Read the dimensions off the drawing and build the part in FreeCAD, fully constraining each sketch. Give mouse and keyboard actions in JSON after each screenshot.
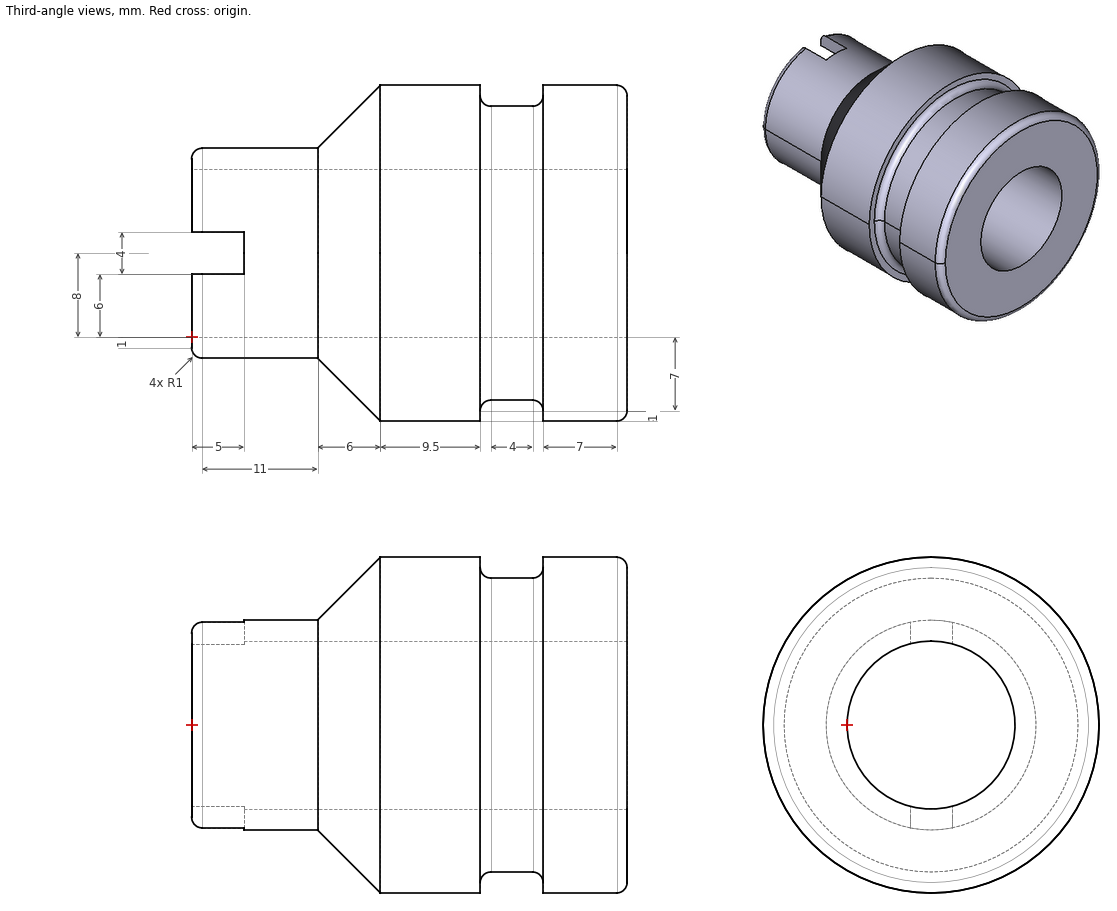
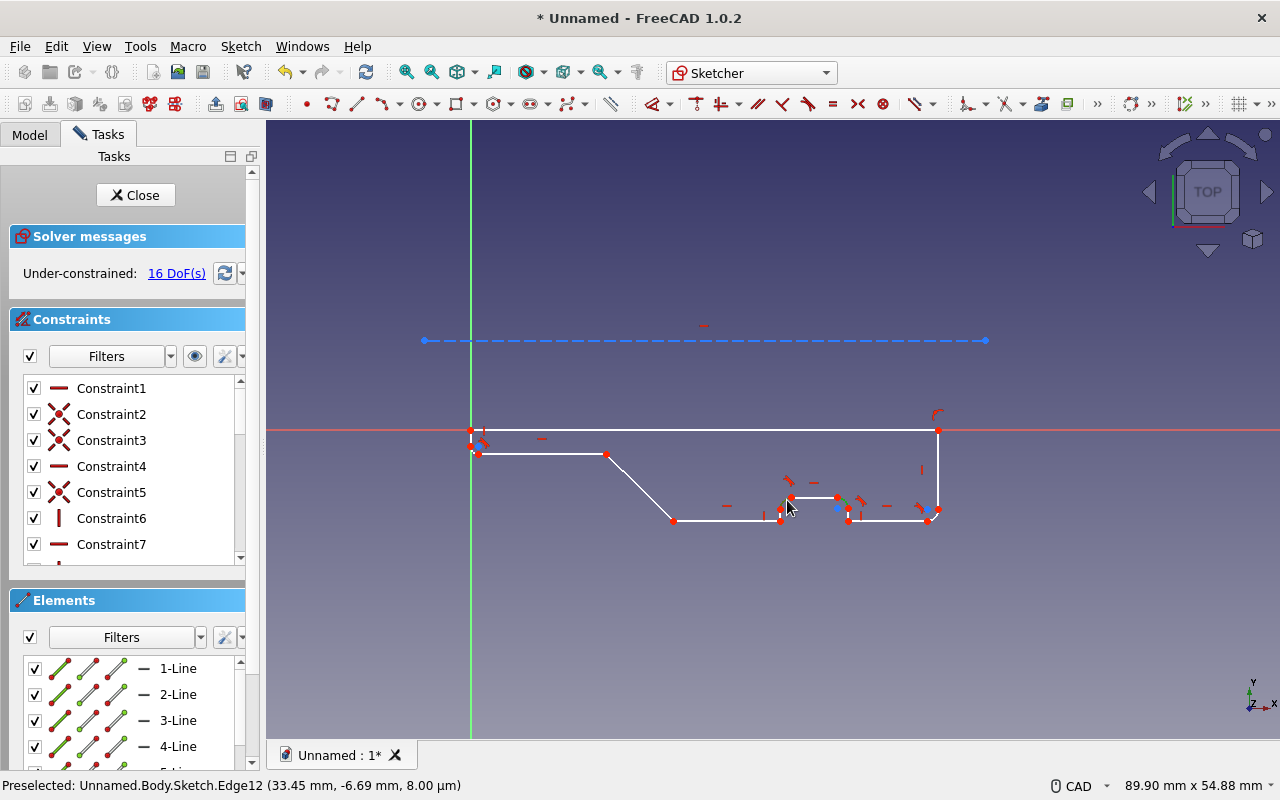
{"action": "scroll", "coordinate": [932, 520], "scroll_direction": "up", "scroll_amount": 5}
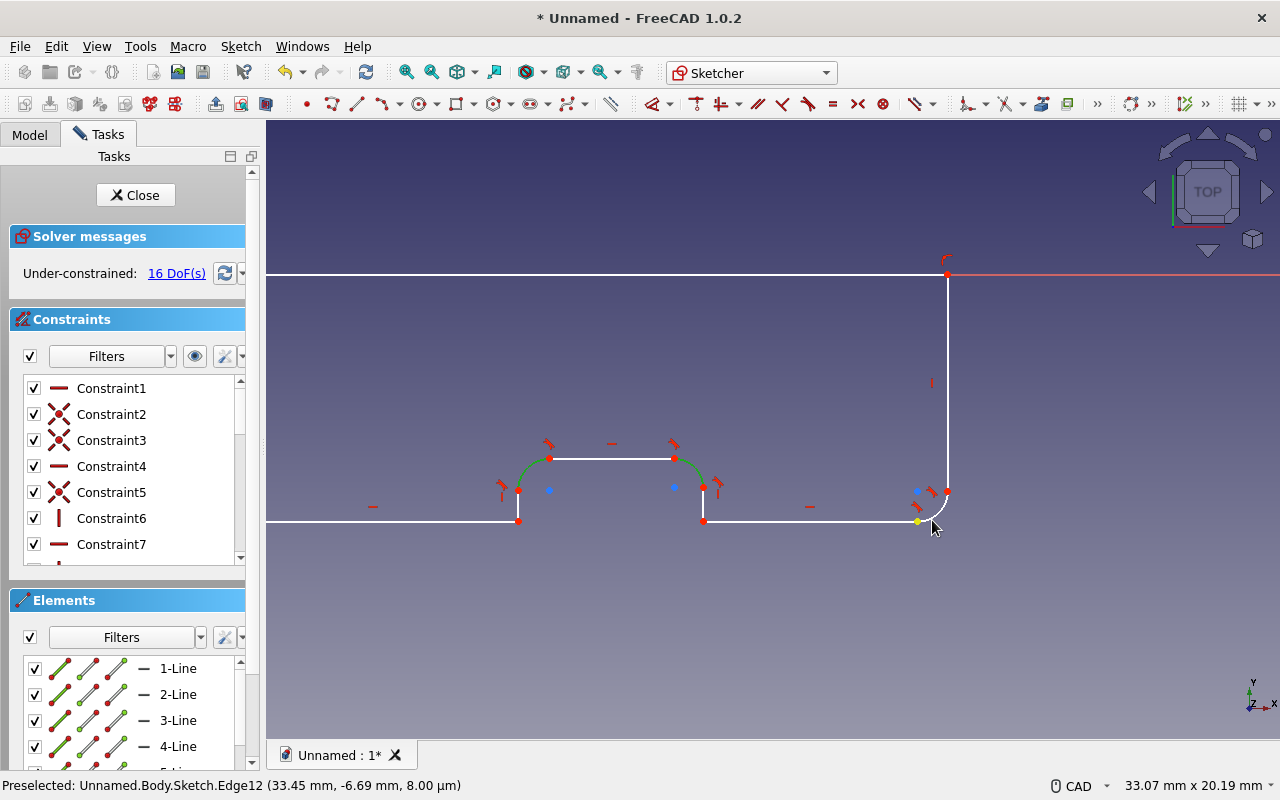
{"action": "left_click", "coordinate": [931, 518]}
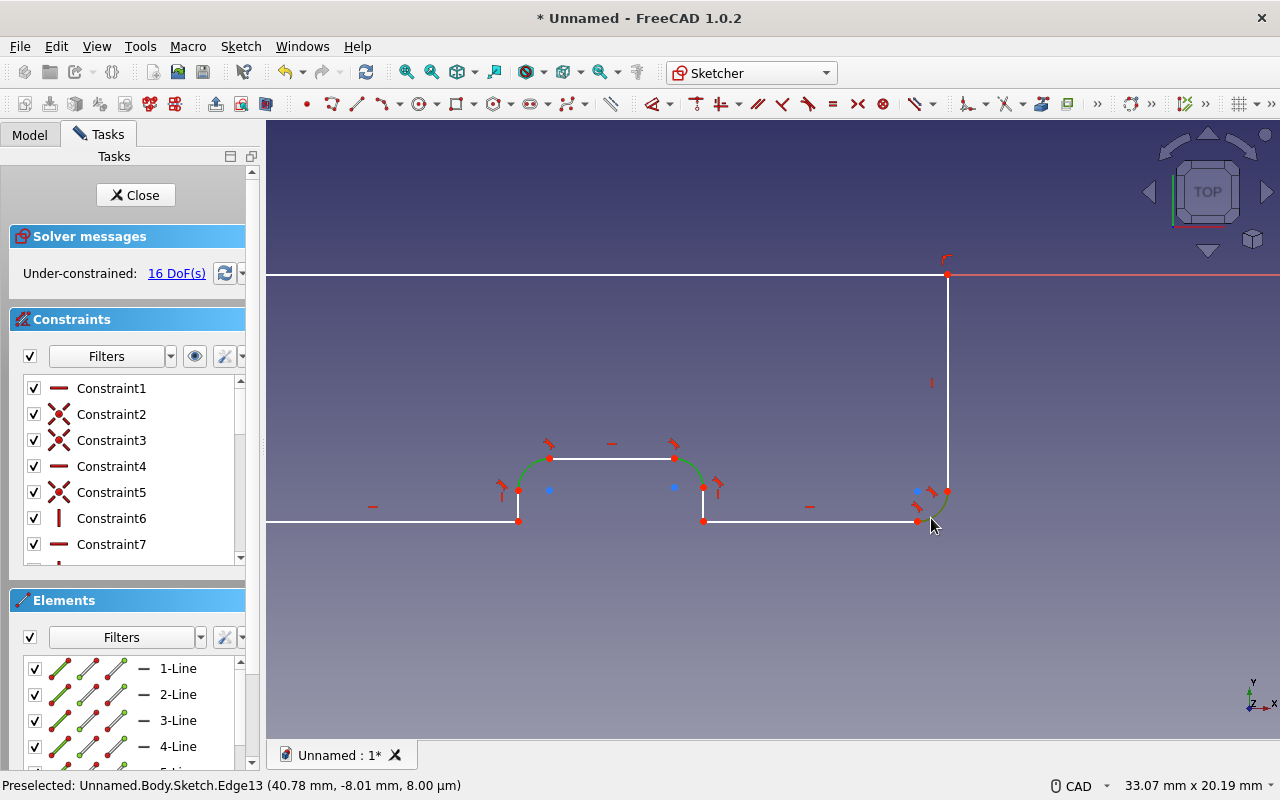
{"action": "scroll", "coordinate": [932, 520], "scroll_direction": "down", "scroll_amount": 5}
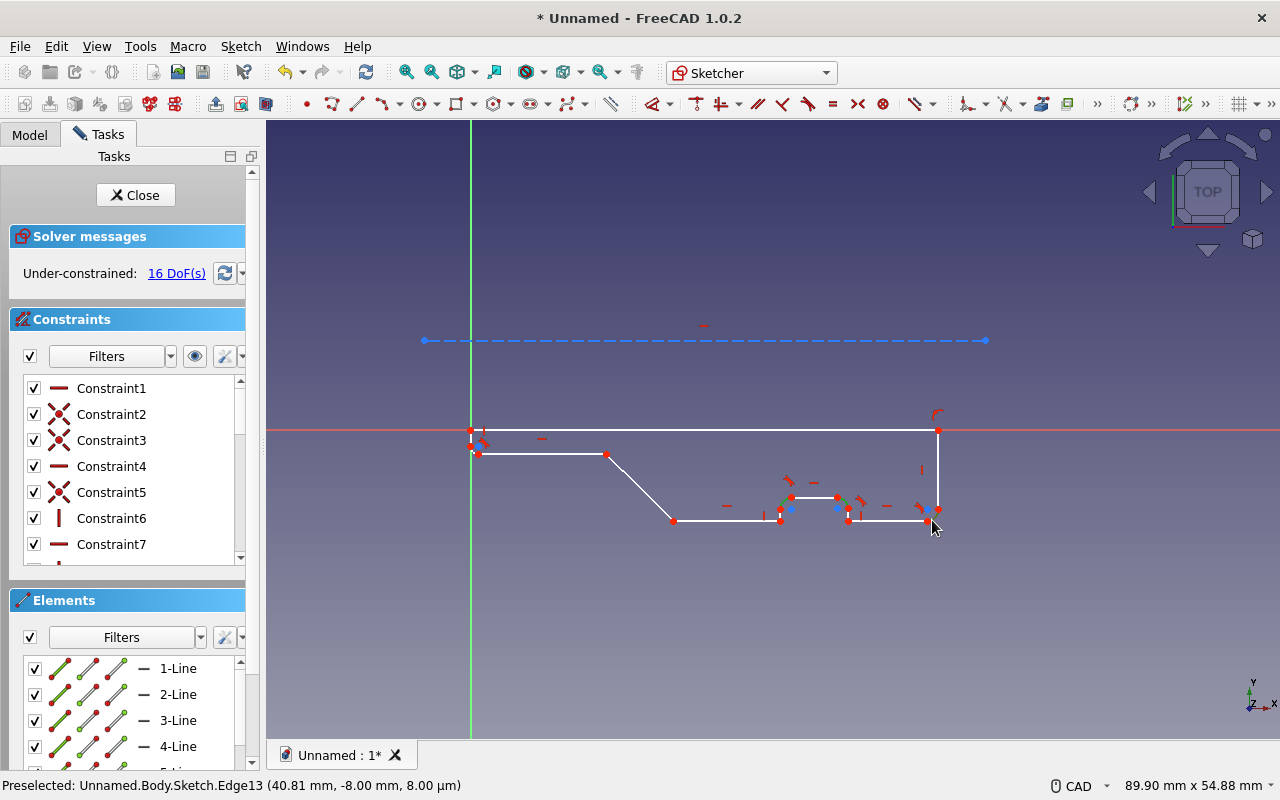
{"action": "scroll", "coordinate": [471, 450], "scroll_direction": "up", "scroll_amount": 7}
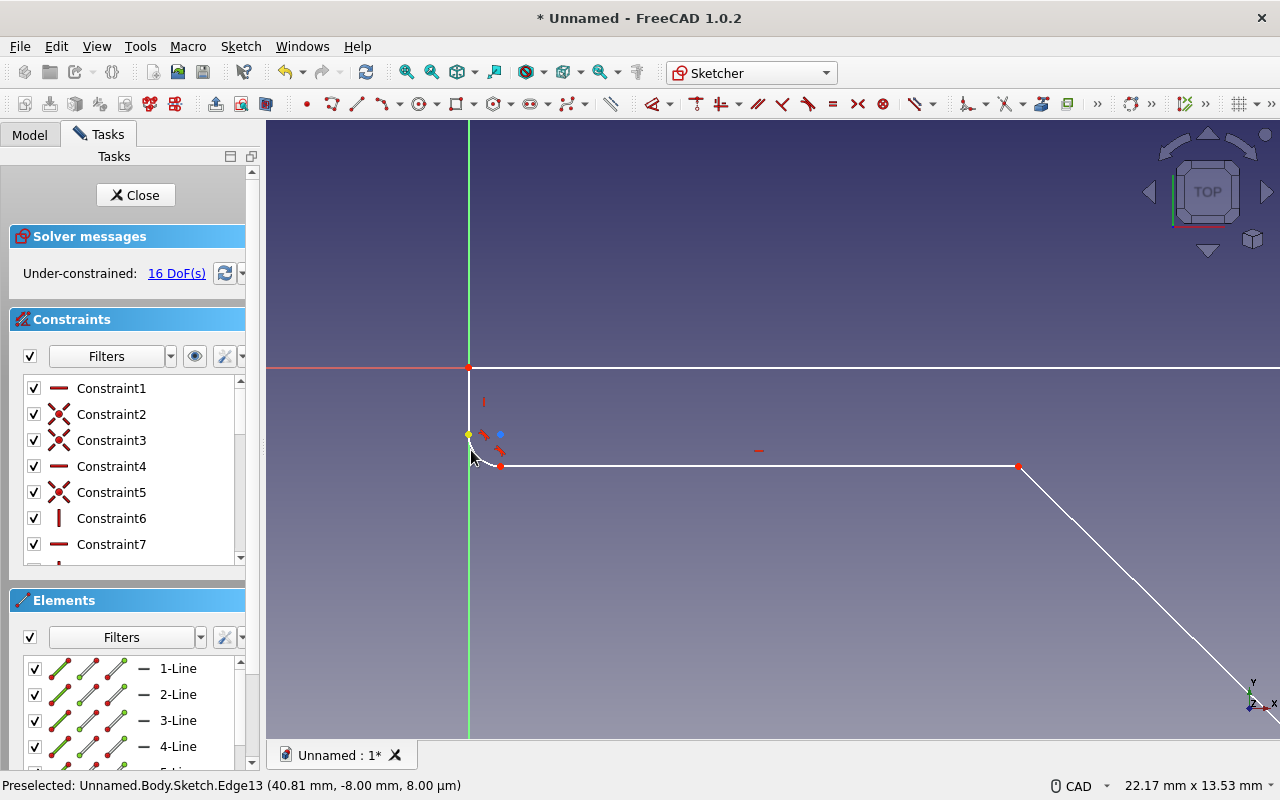
{"action": "left_click", "coordinate": [472, 449]}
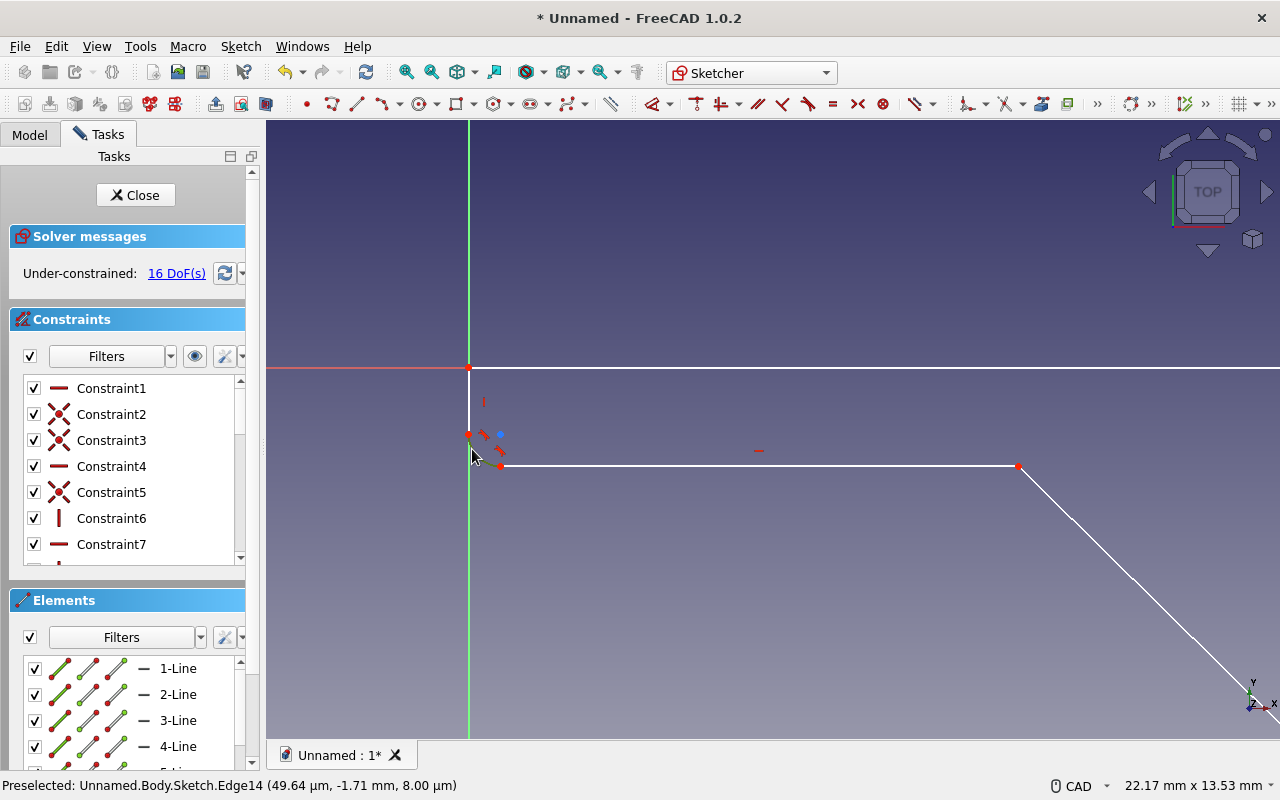
{"action": "key", "text": "e"}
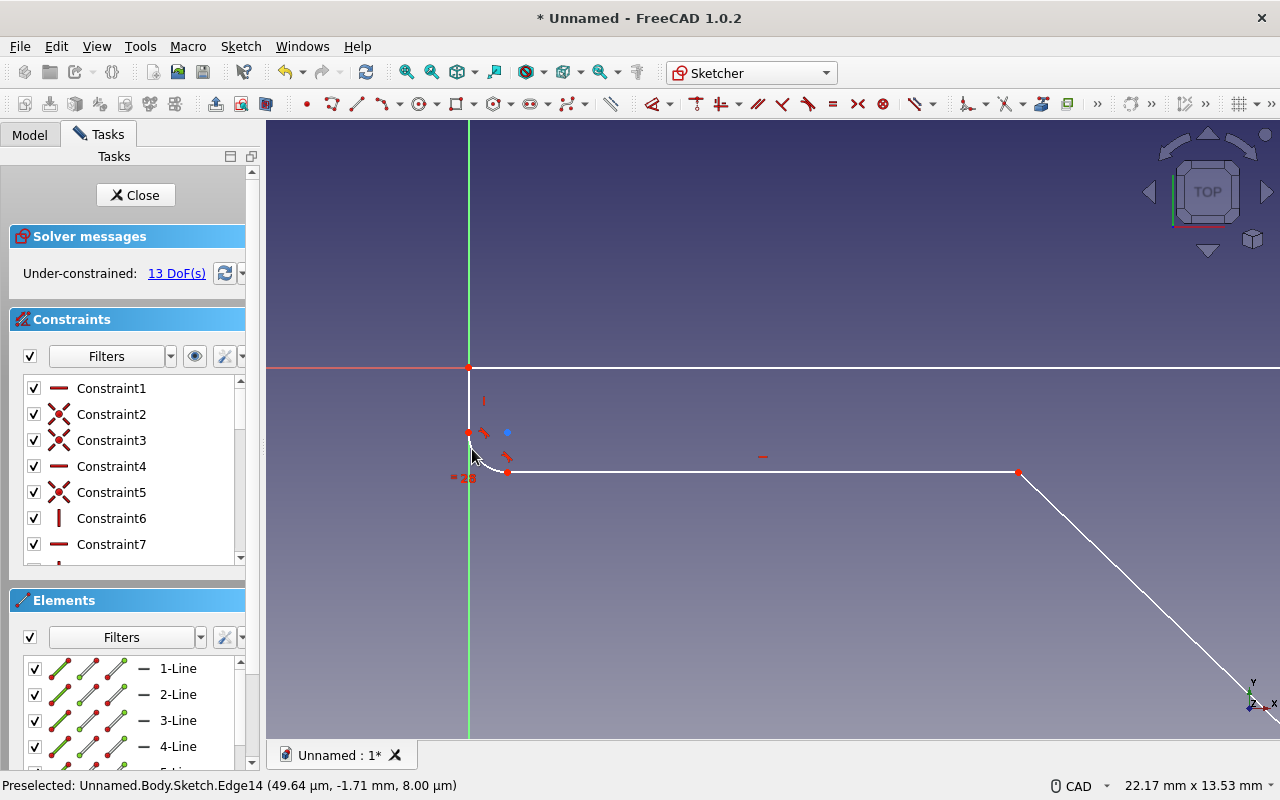
{"action": "left_click", "coordinate": [652, 104]}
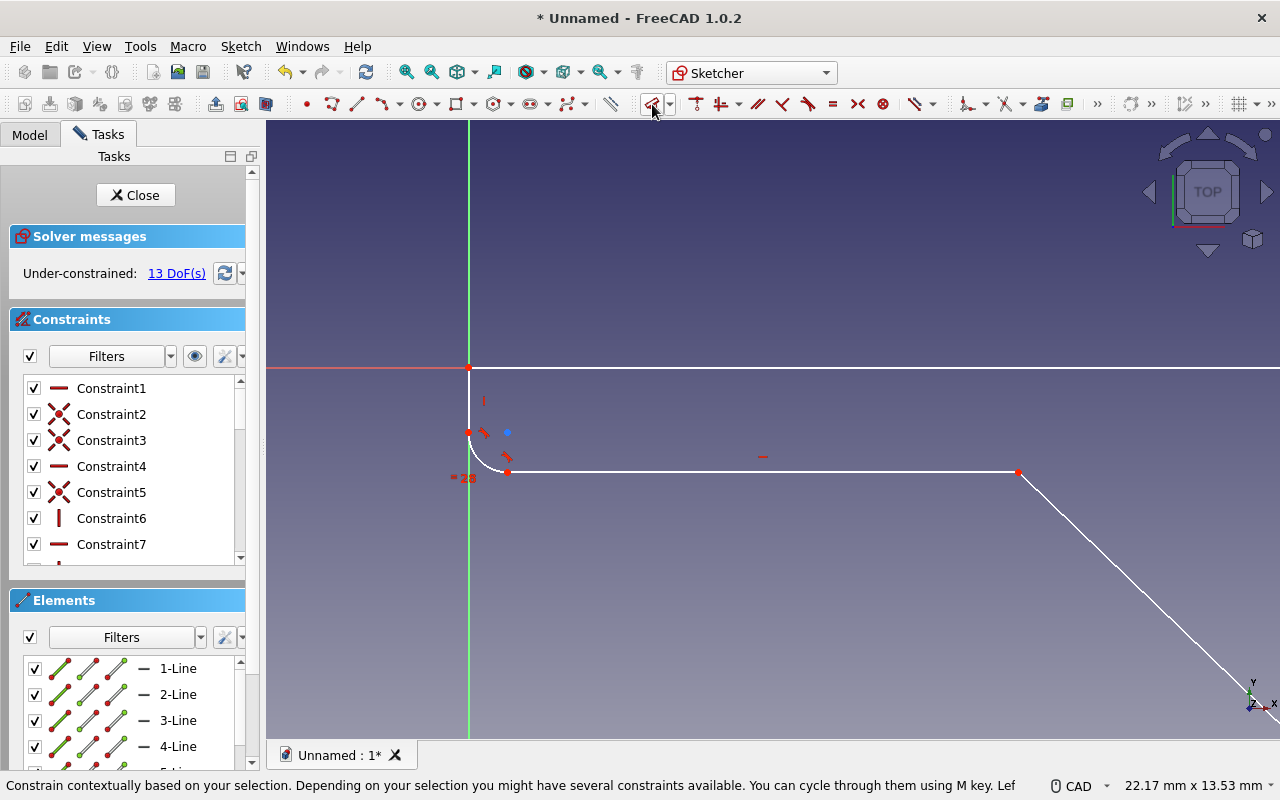
{"action": "scroll", "coordinate": [471, 450], "scroll_direction": "down", "scroll_amount": 7}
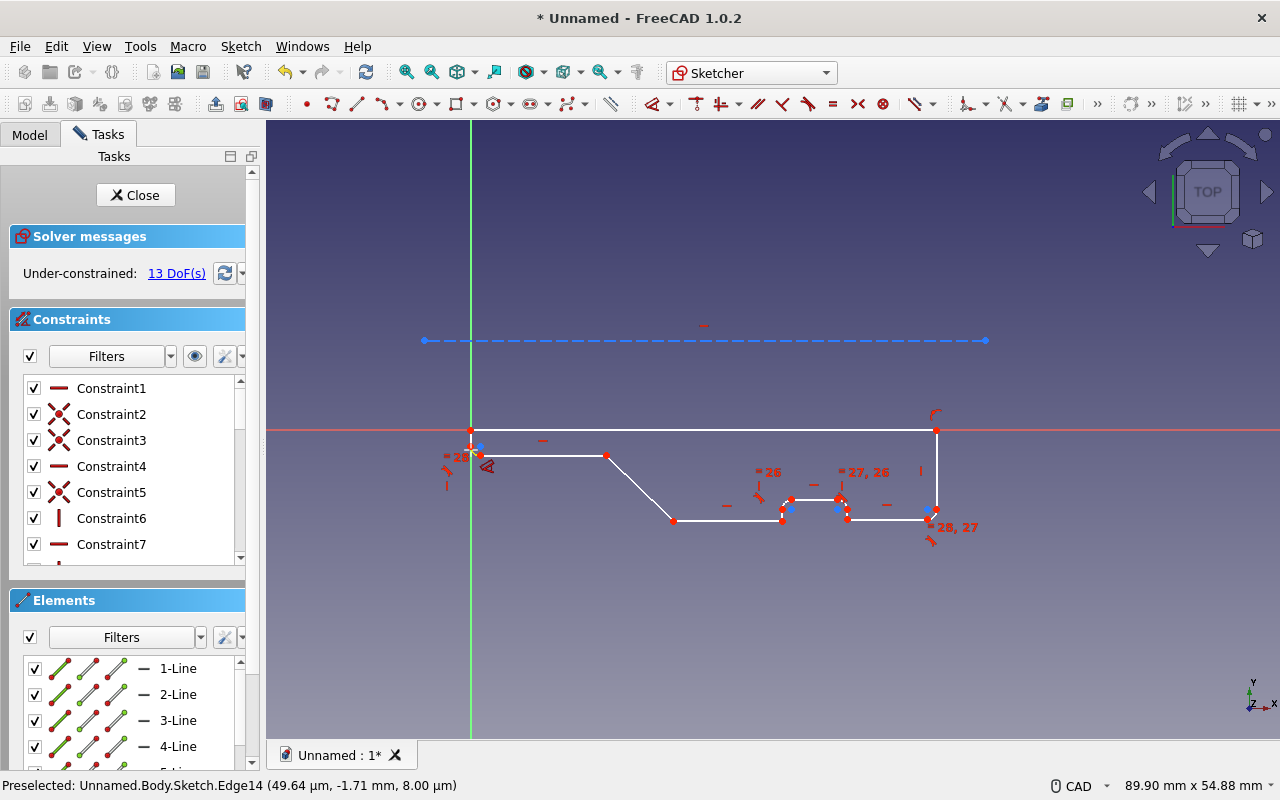
{"action": "scroll", "coordinate": [787, 501], "scroll_direction": "up", "scroll_amount": 7}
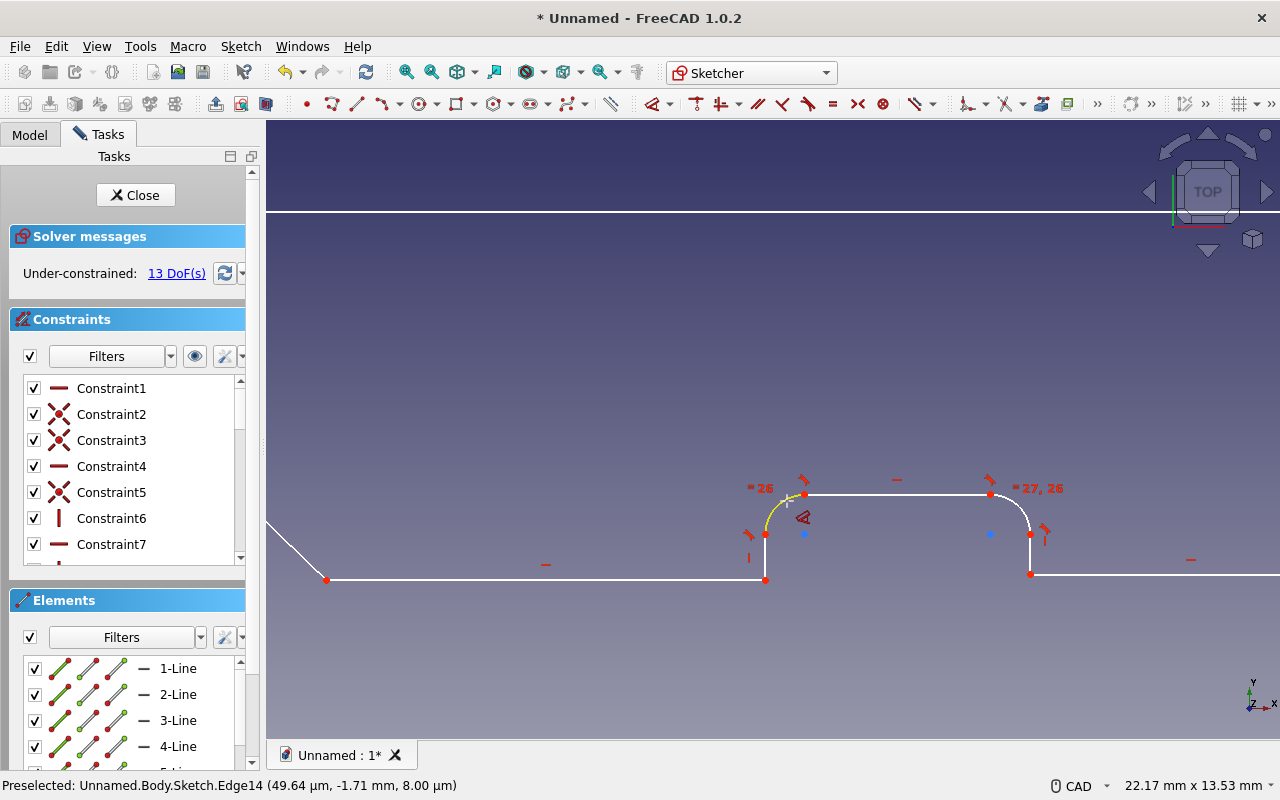
{"action": "left_click", "coordinate": [787, 499]}
{"action": "left_click", "coordinate": [773, 470]}